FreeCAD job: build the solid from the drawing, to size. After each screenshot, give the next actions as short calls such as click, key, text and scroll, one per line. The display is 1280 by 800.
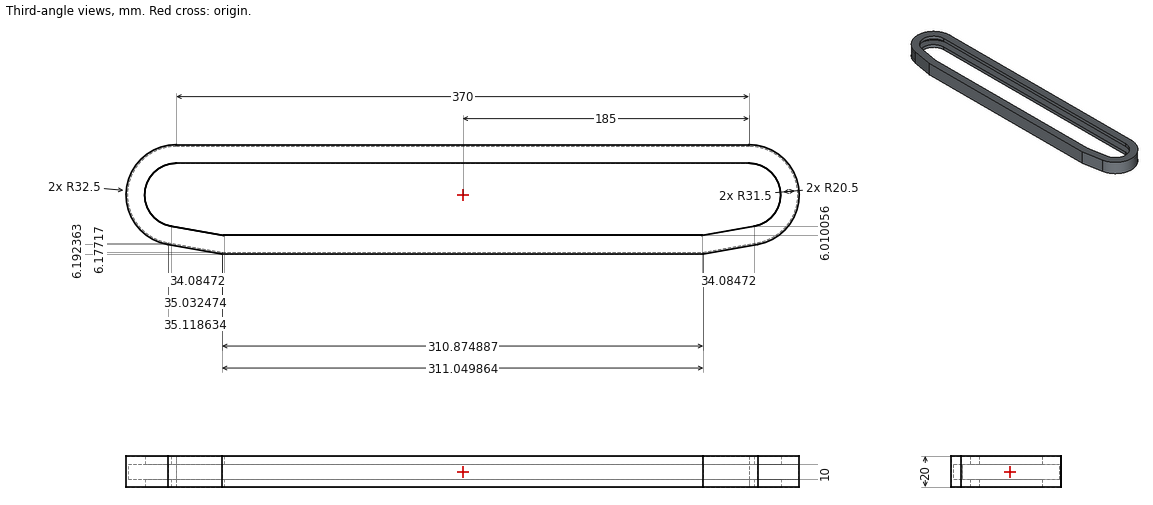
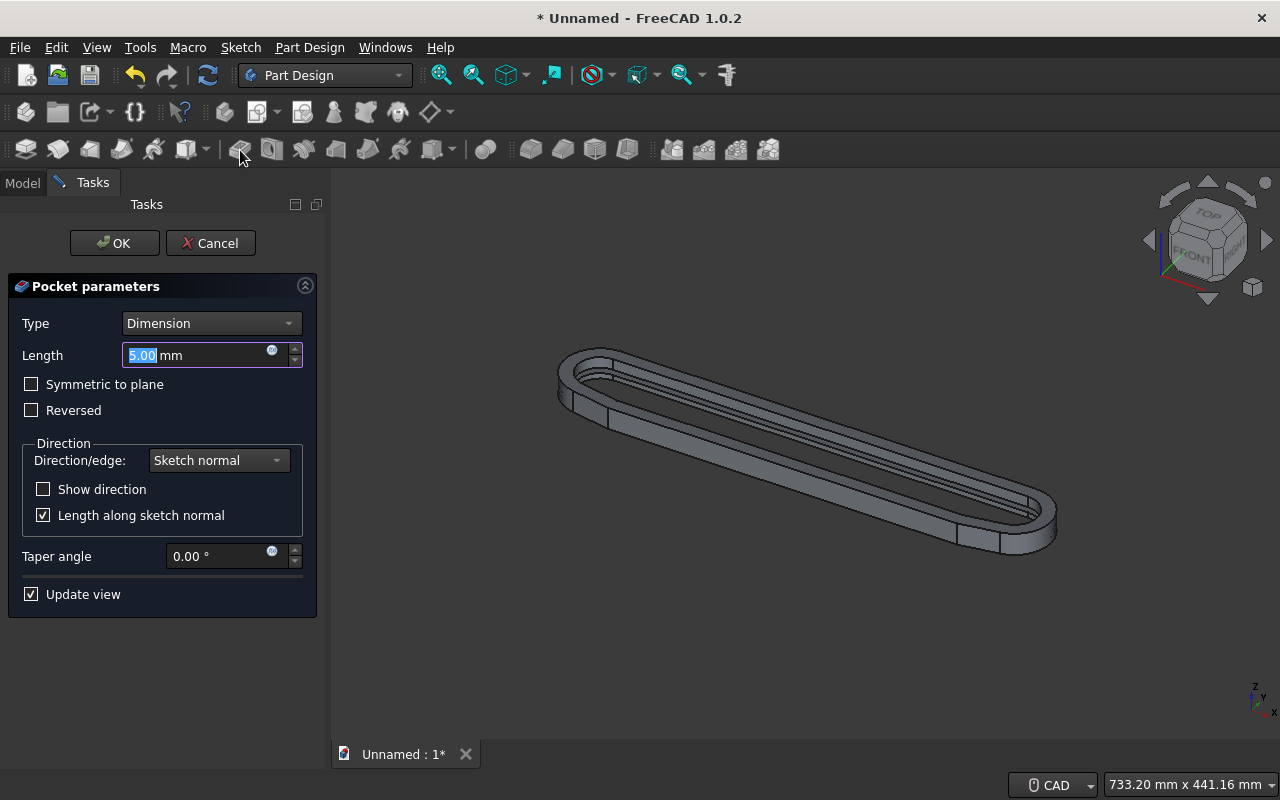
text(10)
key(Tab)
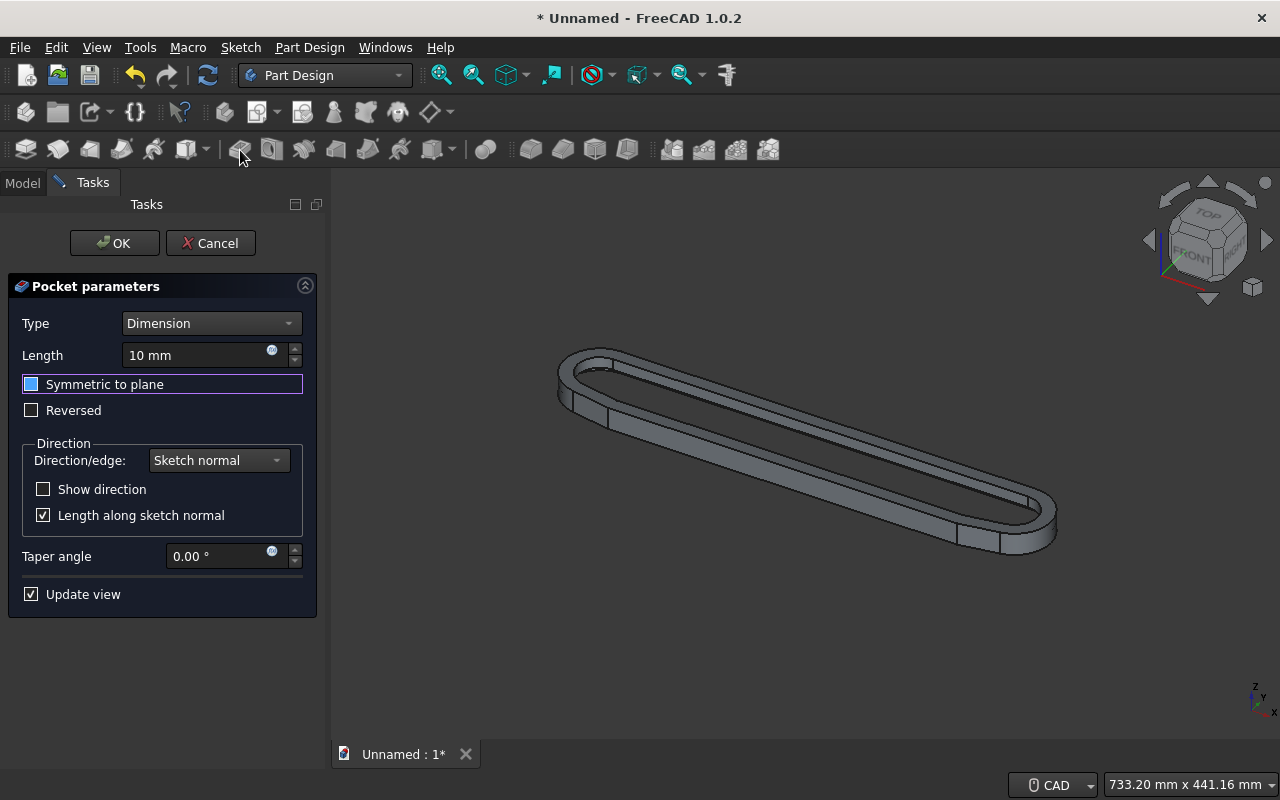
click(30, 384)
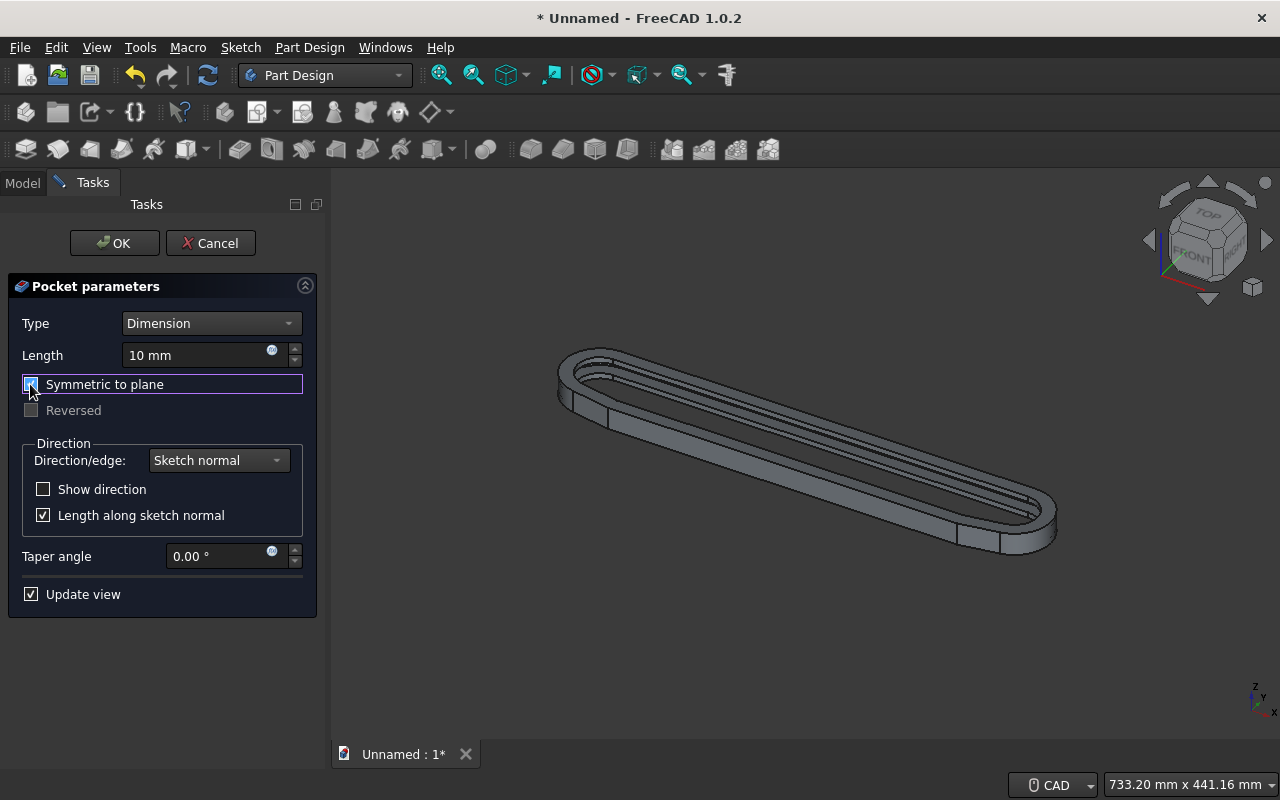
click(115, 243)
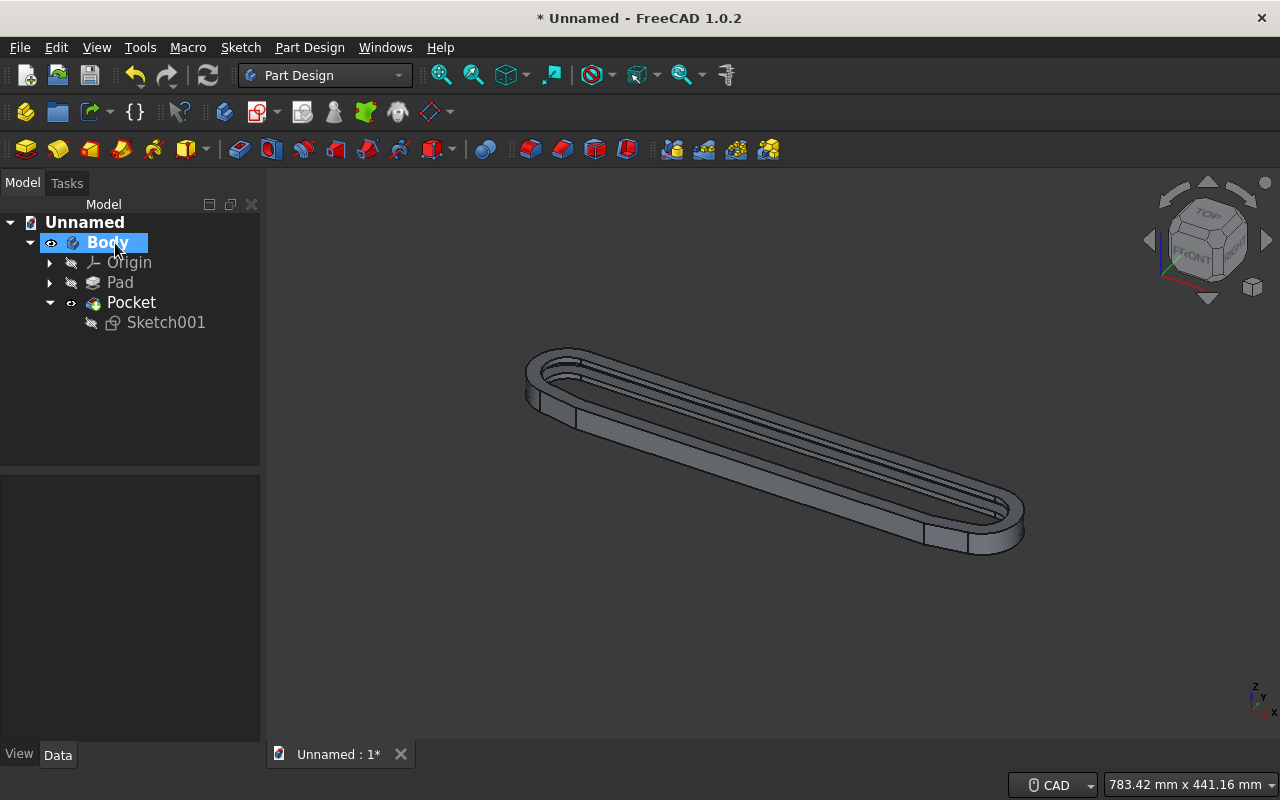
key(0)